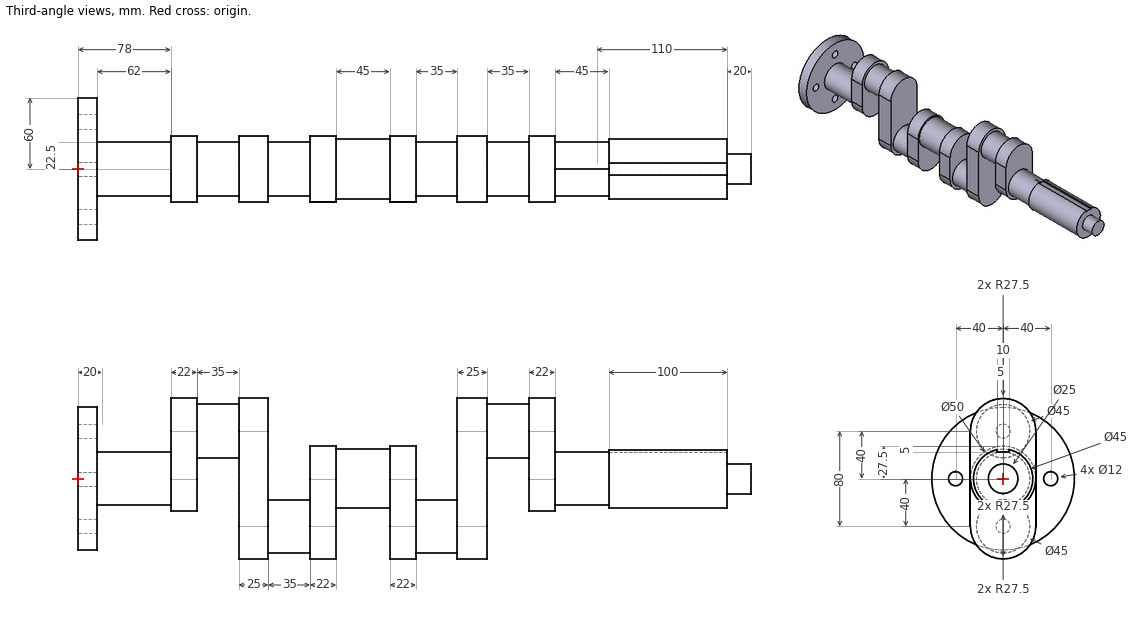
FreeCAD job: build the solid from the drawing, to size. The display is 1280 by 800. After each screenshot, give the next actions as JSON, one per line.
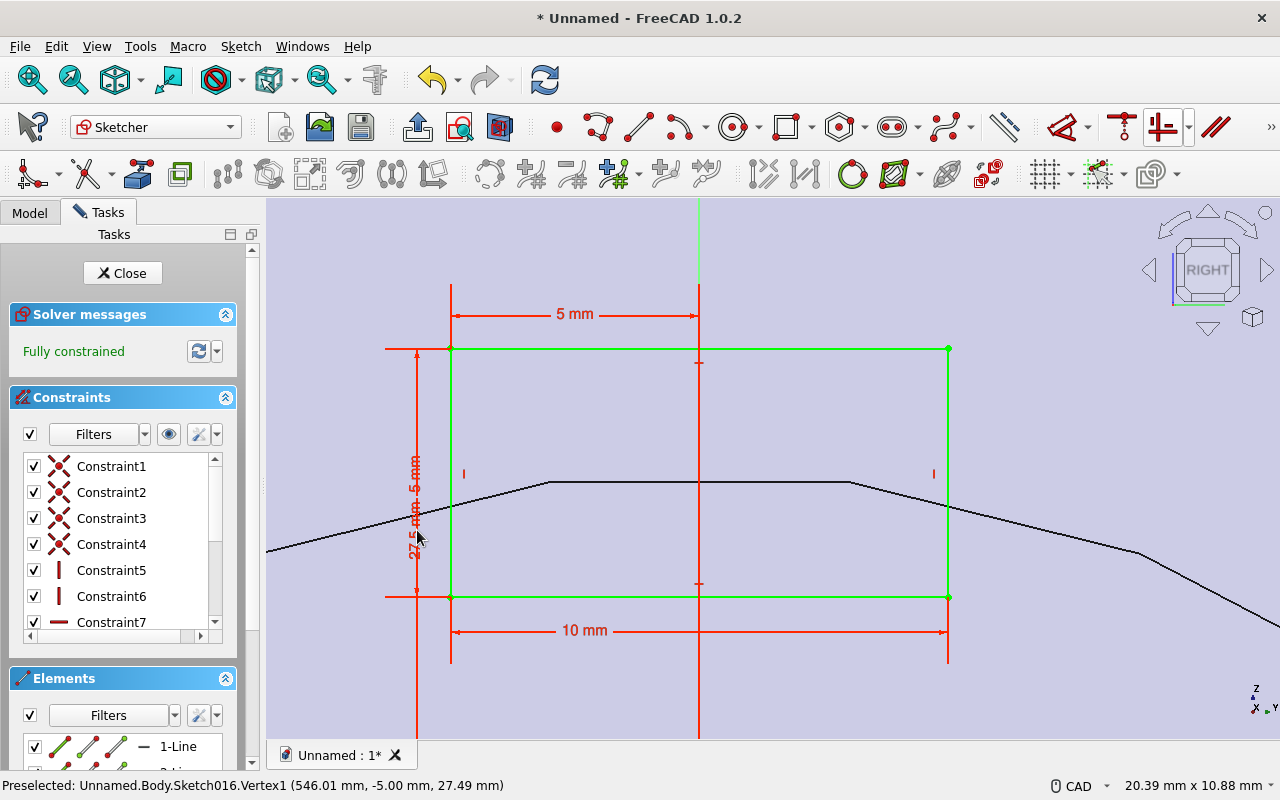
{"action": "left_click", "coordinate": [123, 273]}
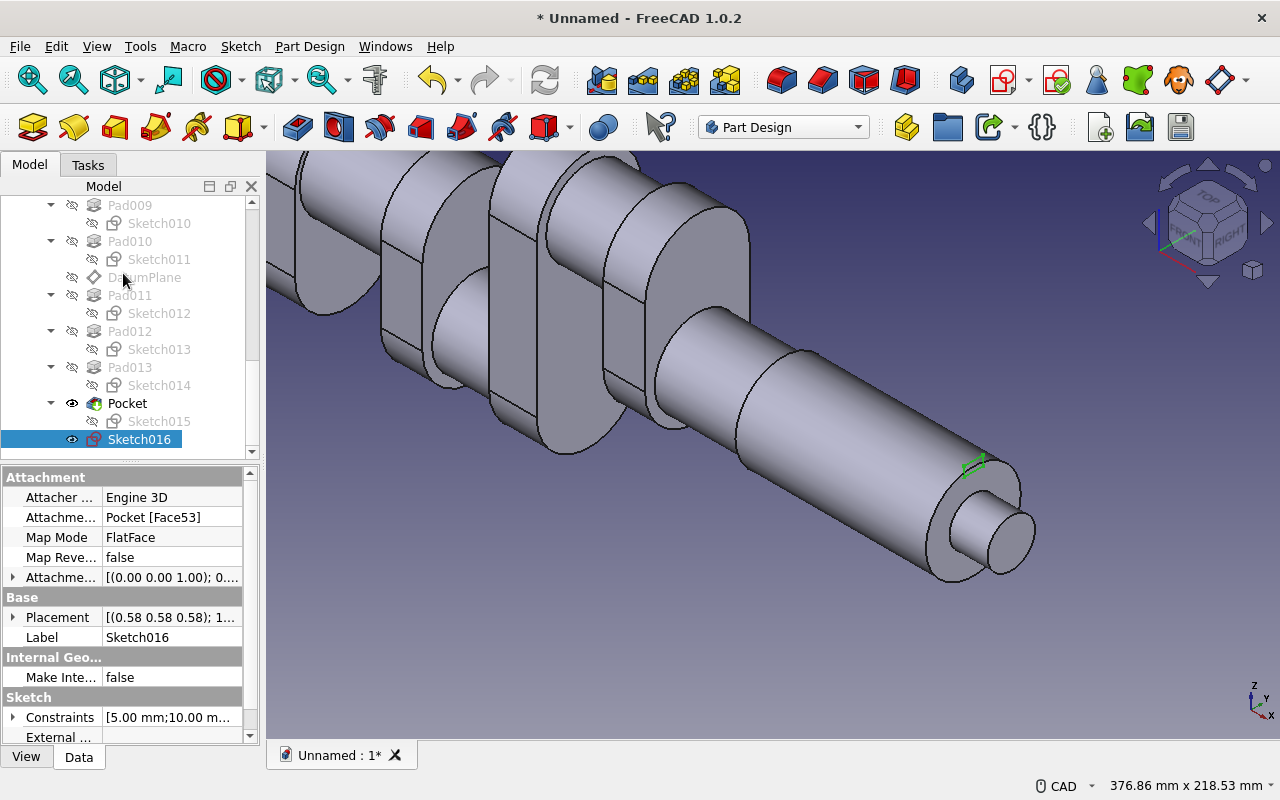
{"action": "left_click", "coordinate": [298, 128]}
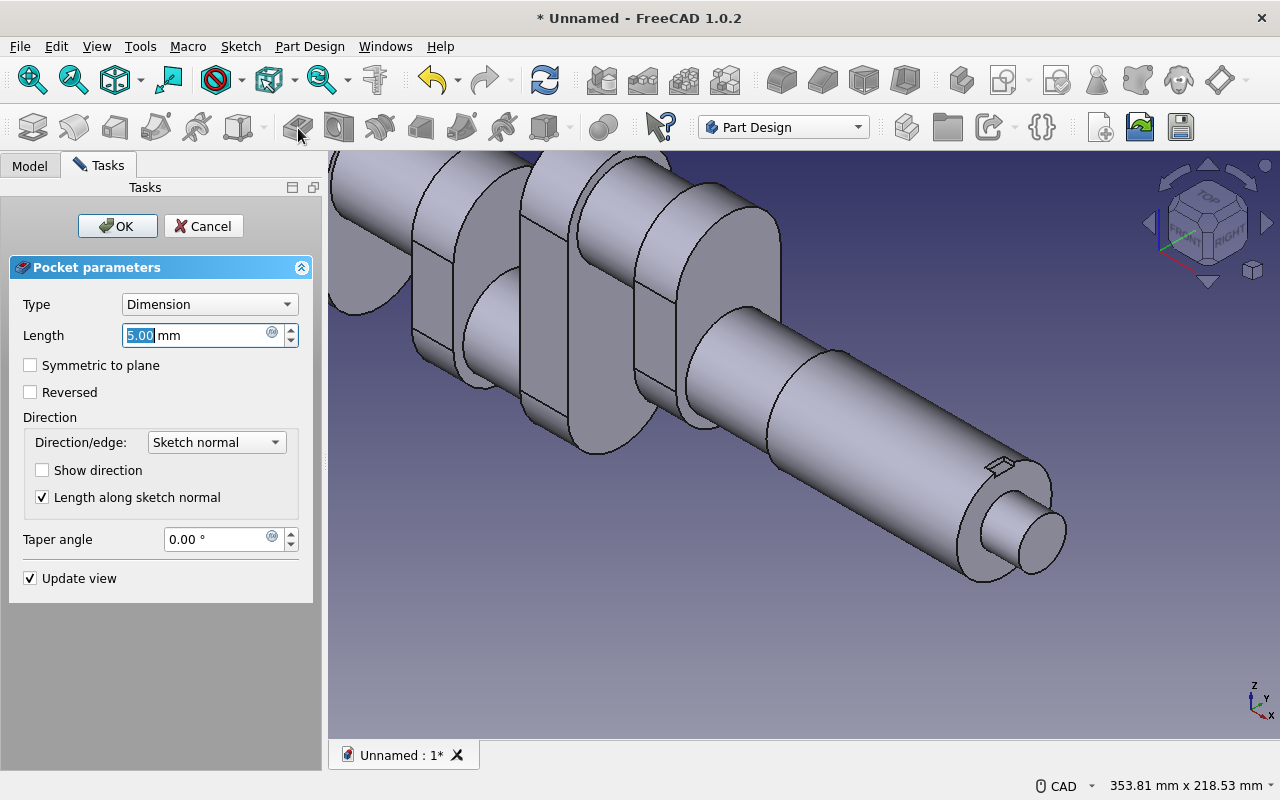
{"action": "type", "text": "110"}
{"action": "key", "text": "Tab"}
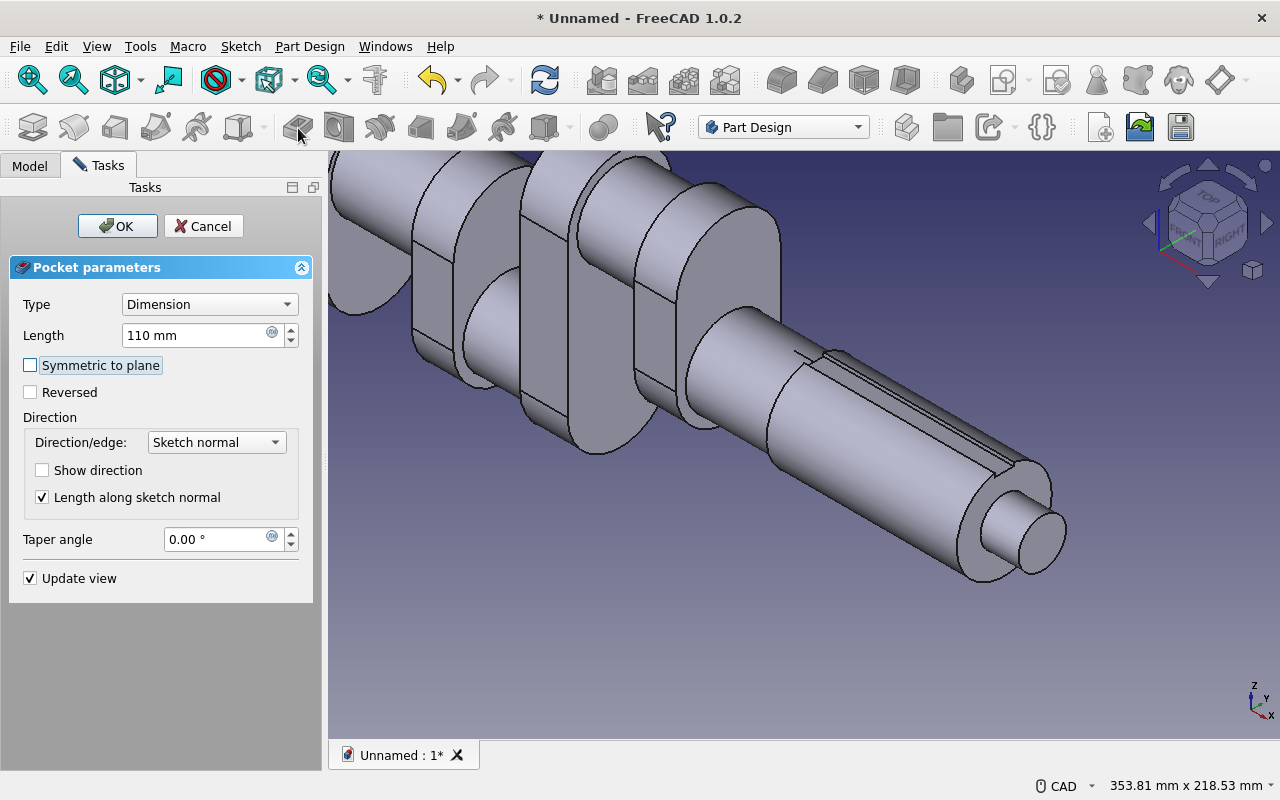
{"action": "left_click", "coordinate": [118, 226]}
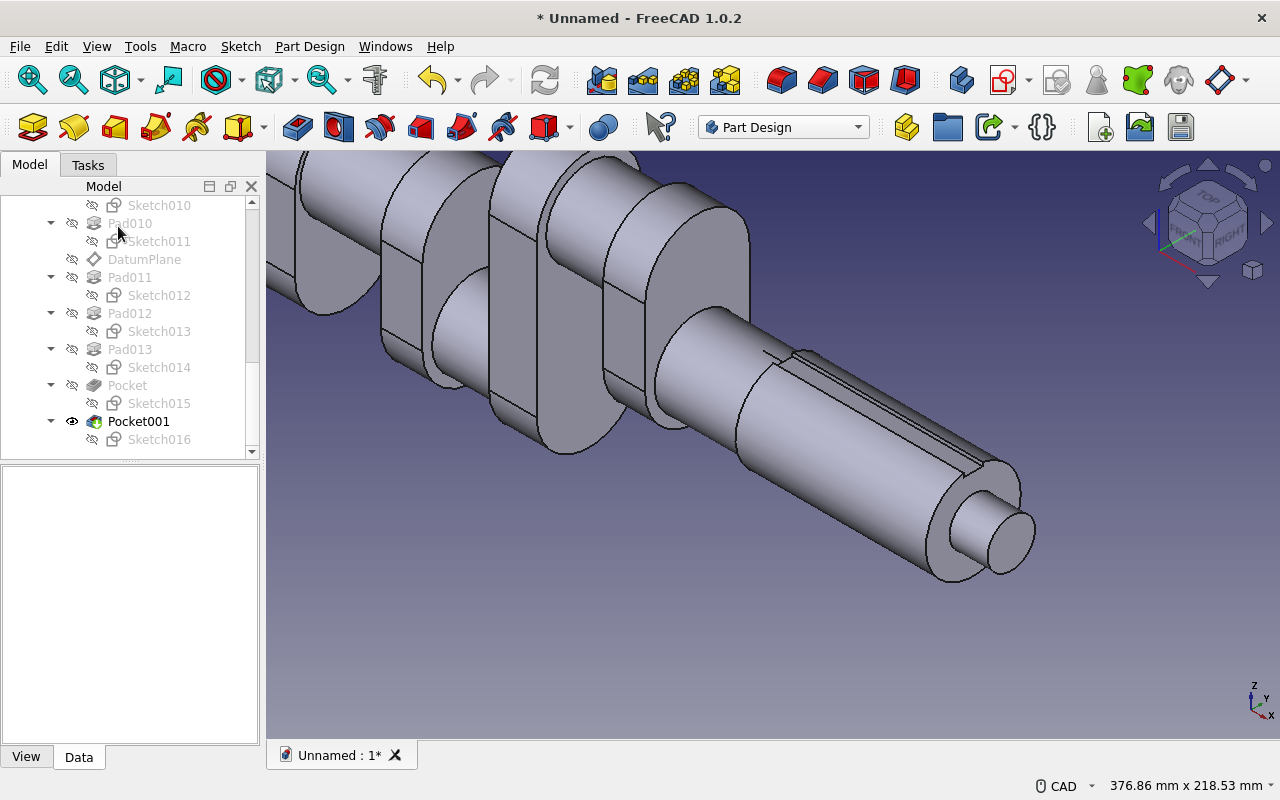
{"action": "left_click", "coordinate": [33, 80]}